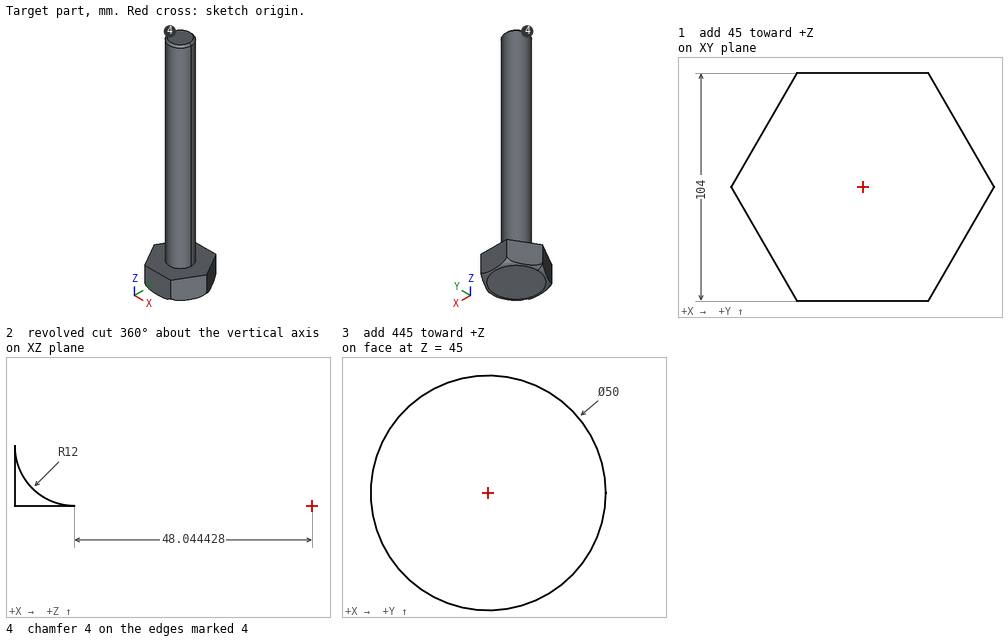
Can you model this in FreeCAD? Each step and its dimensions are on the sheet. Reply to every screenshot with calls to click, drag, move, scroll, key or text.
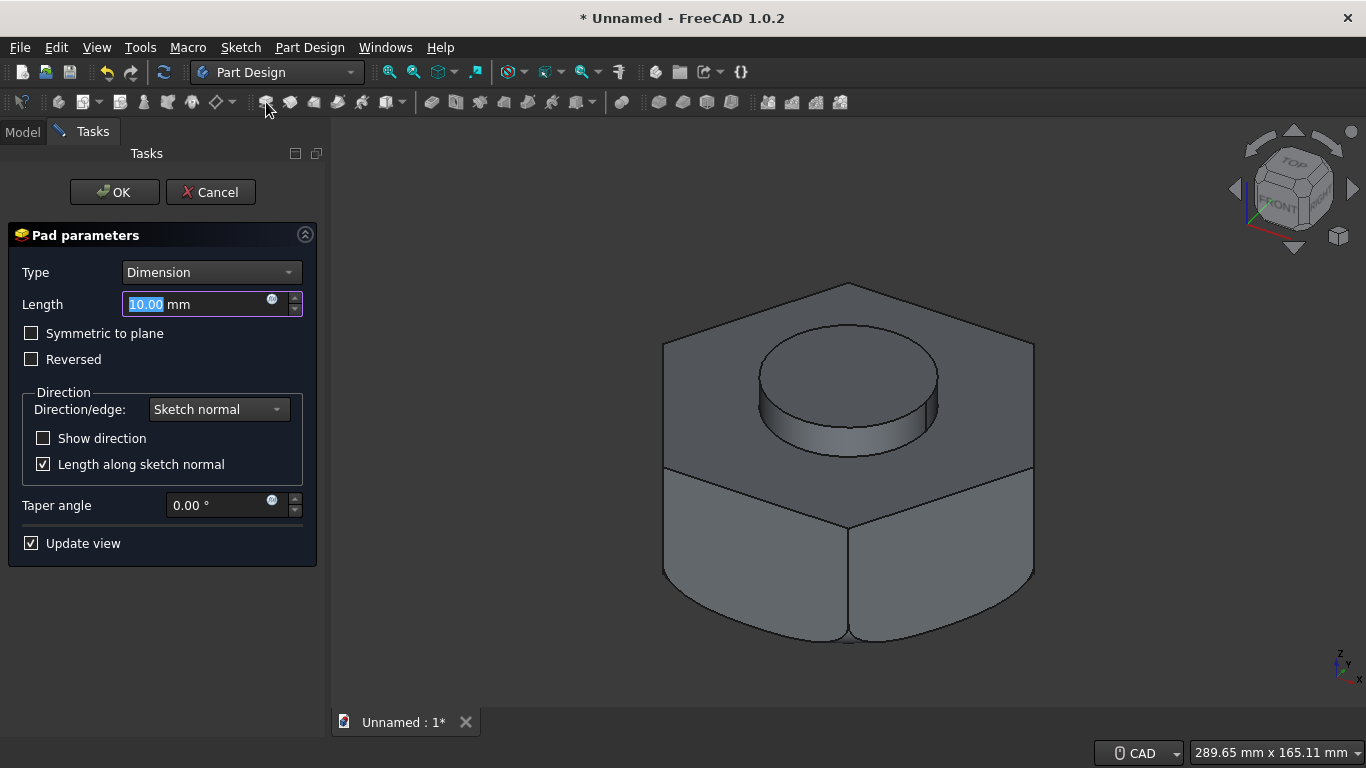
text(445)
key(Tab)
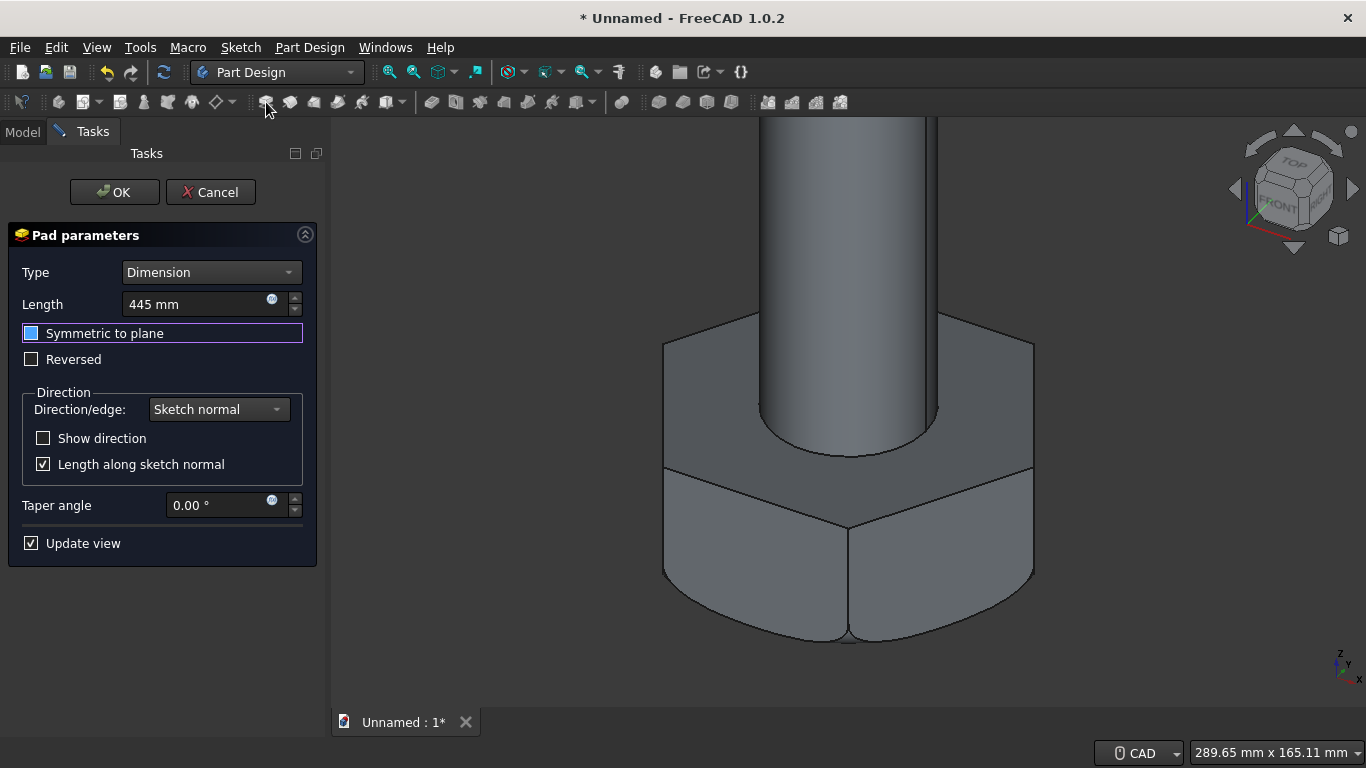
click(115, 192)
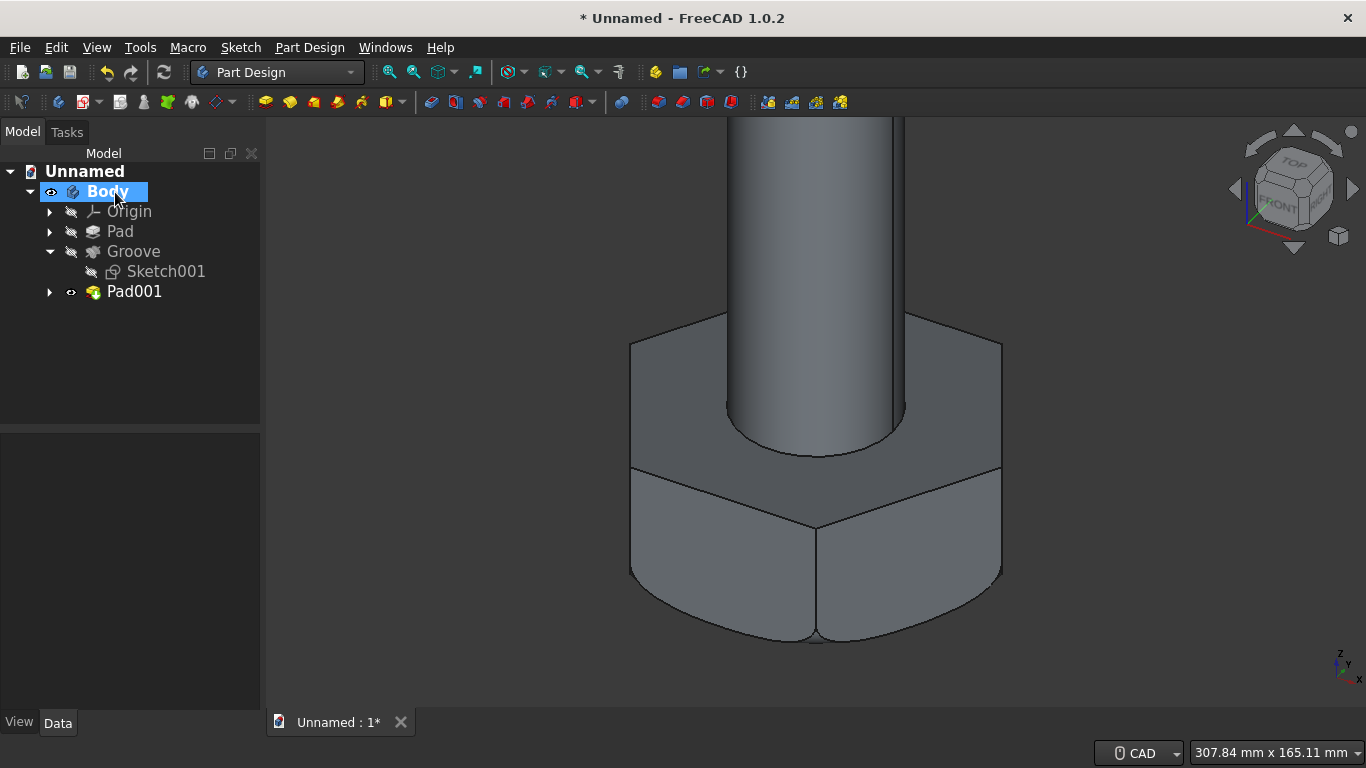
key(v)
key(f)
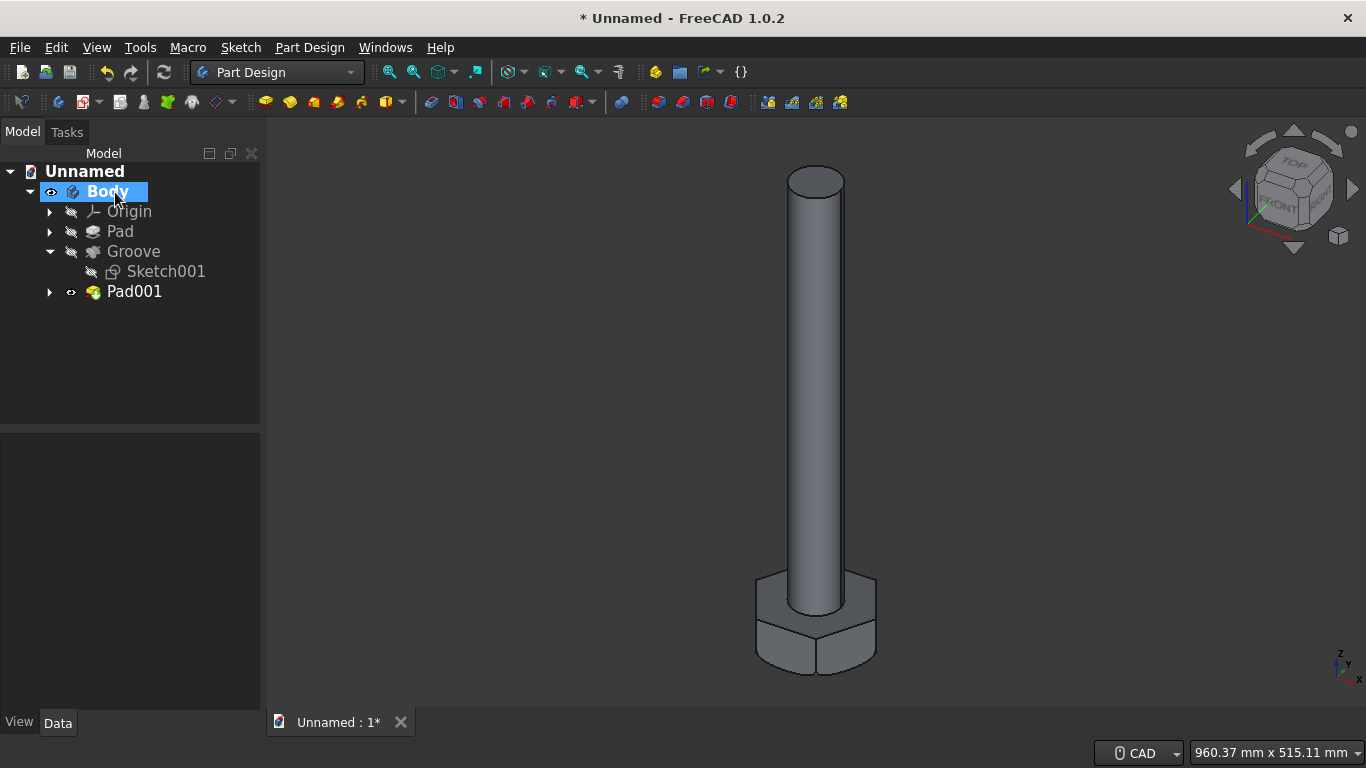
click(804, 166)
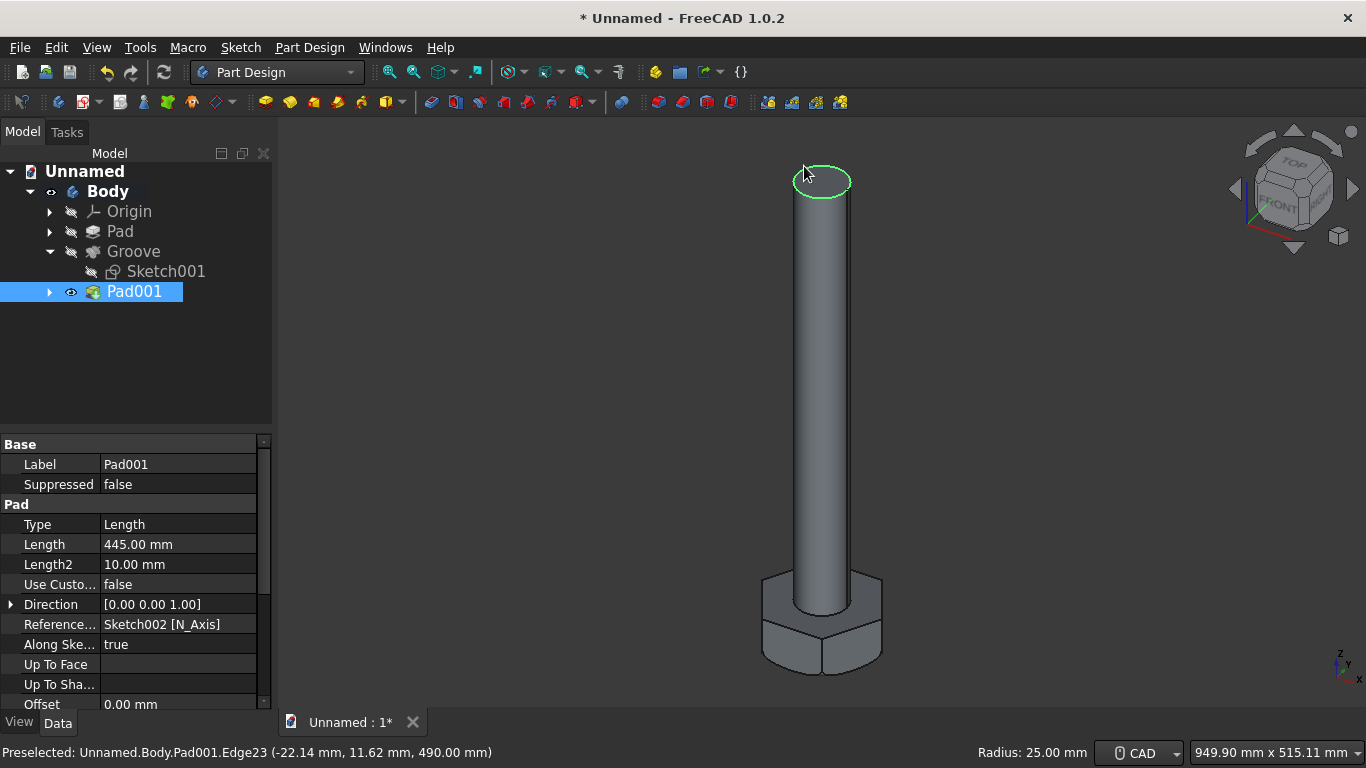
click(684, 102)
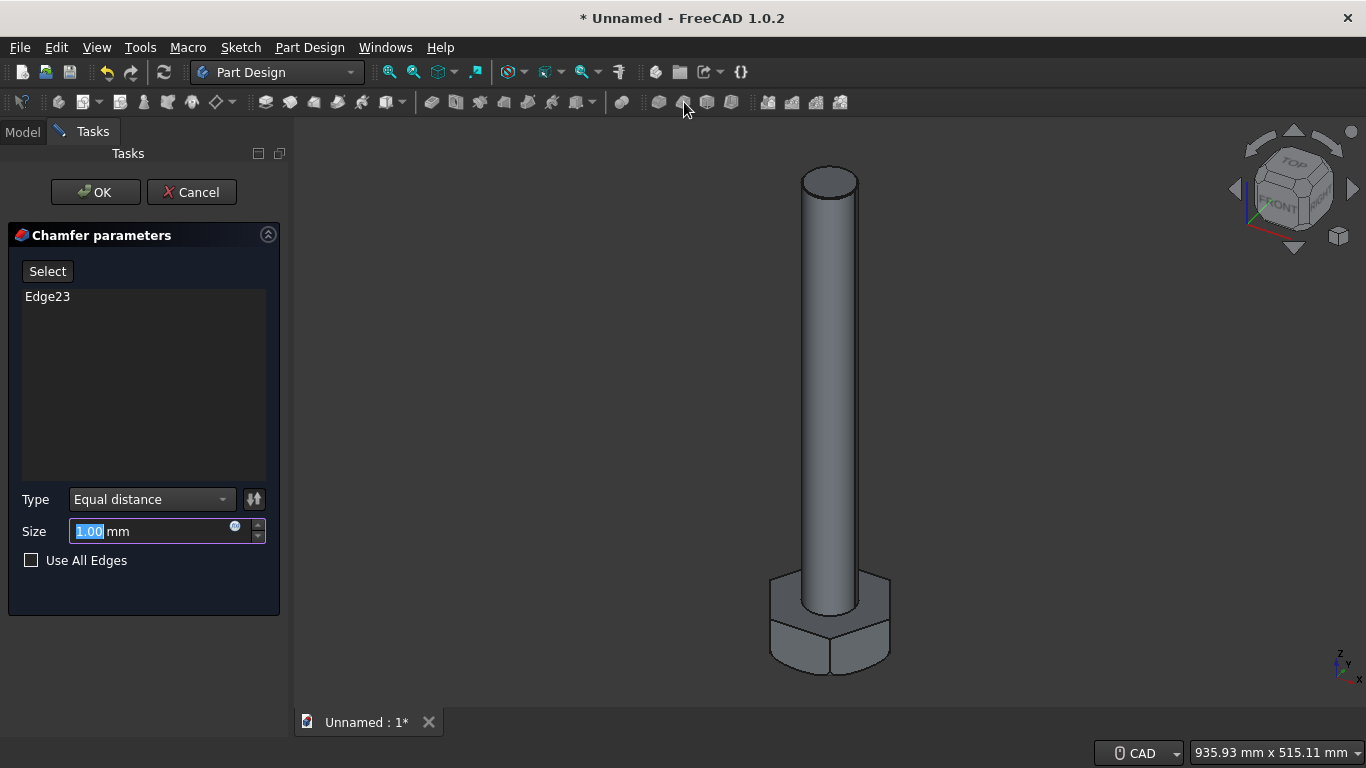
text(4)
key(Tab)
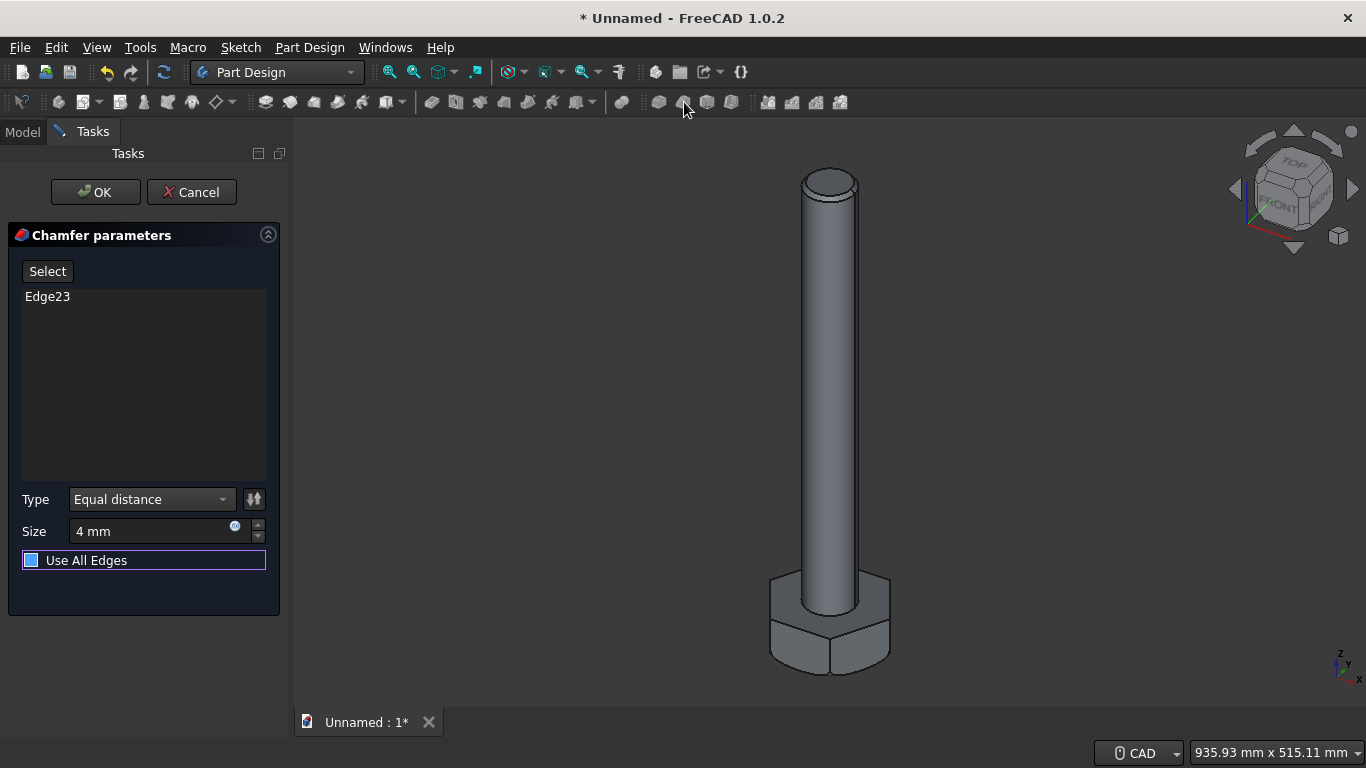
click(96, 192)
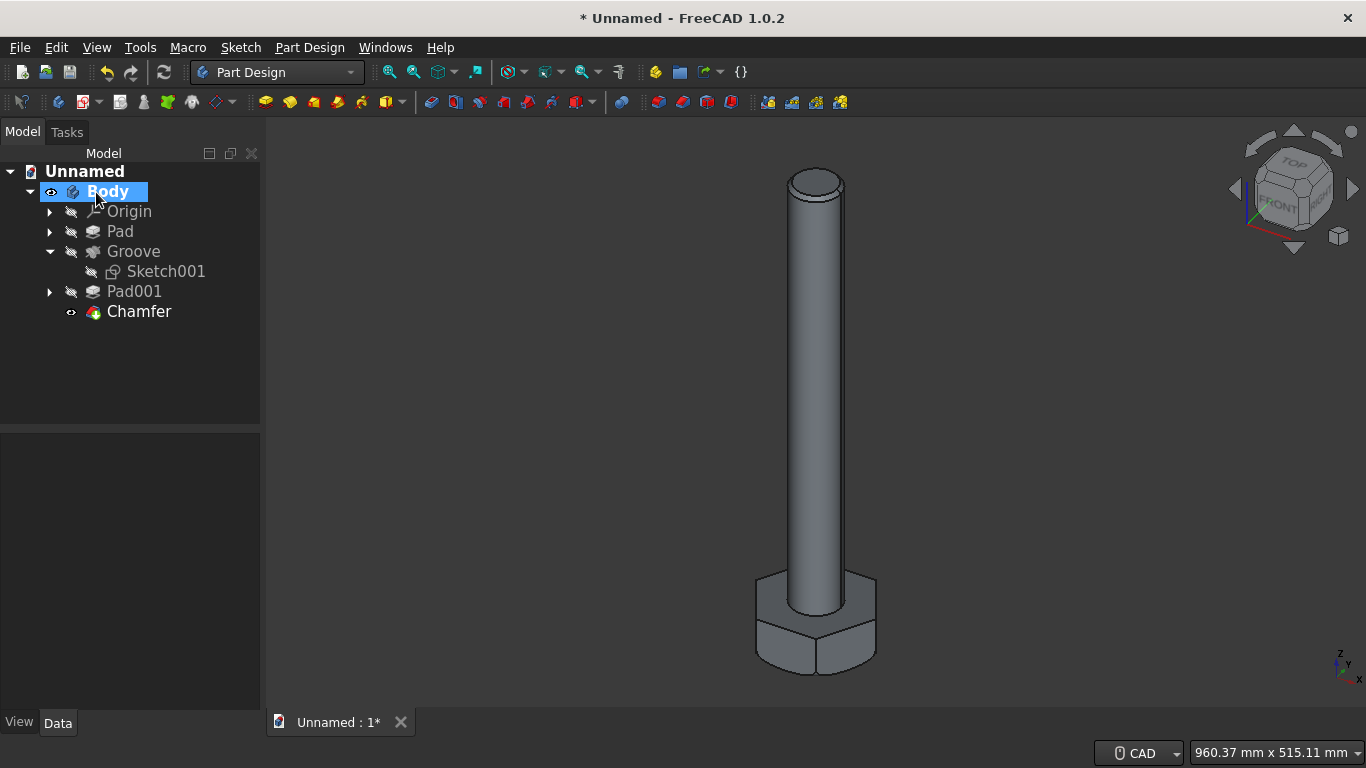
key(0)